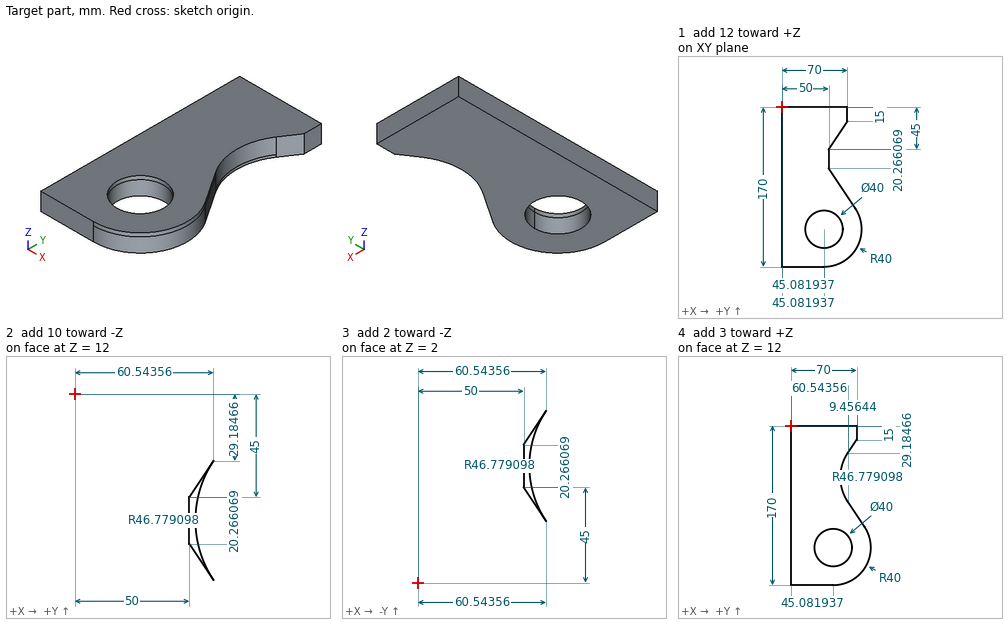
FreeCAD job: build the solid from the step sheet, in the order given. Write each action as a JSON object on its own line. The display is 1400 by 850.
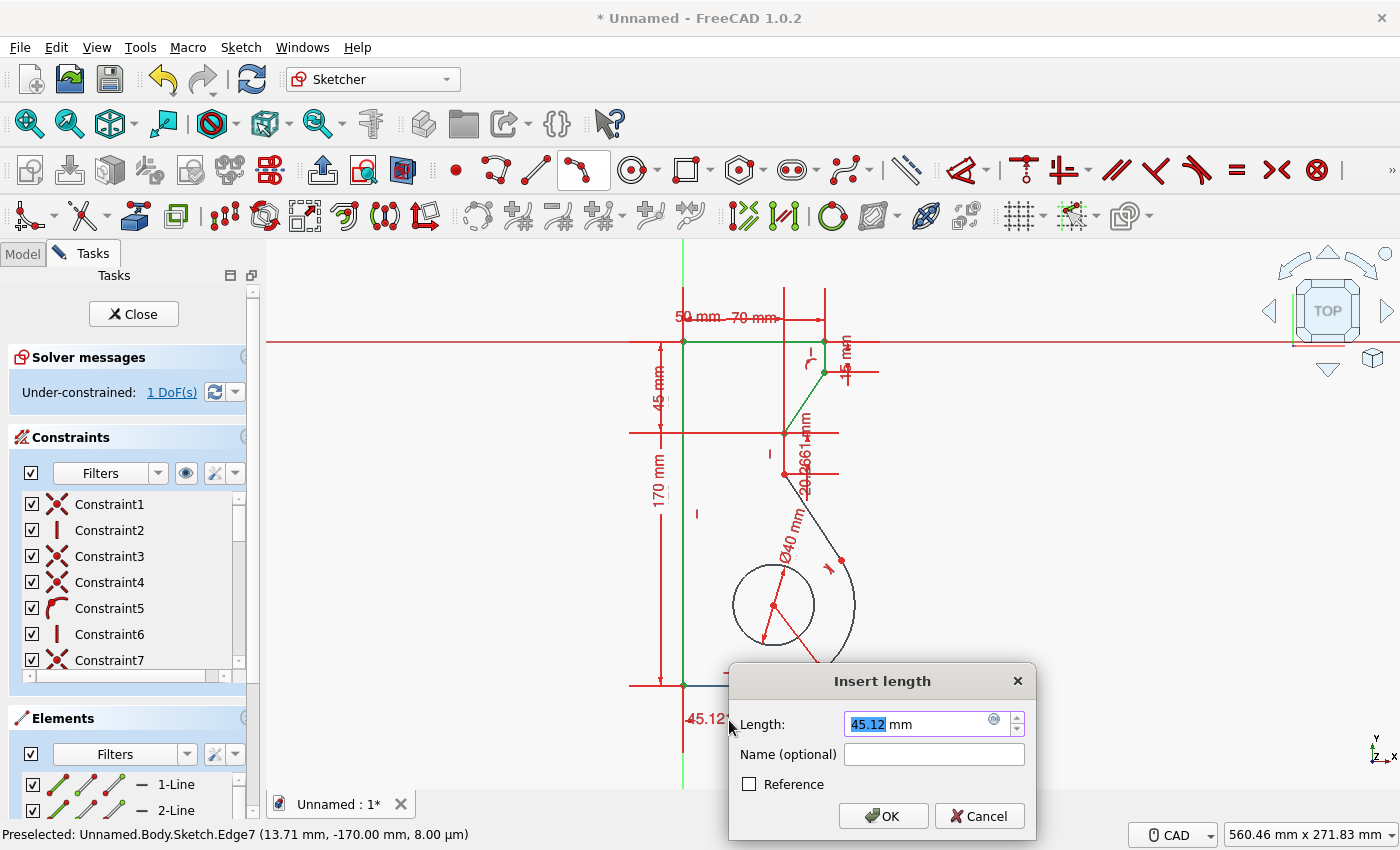
{"action": "type", "text": "45.081937"}
{"action": "key", "text": "Return"}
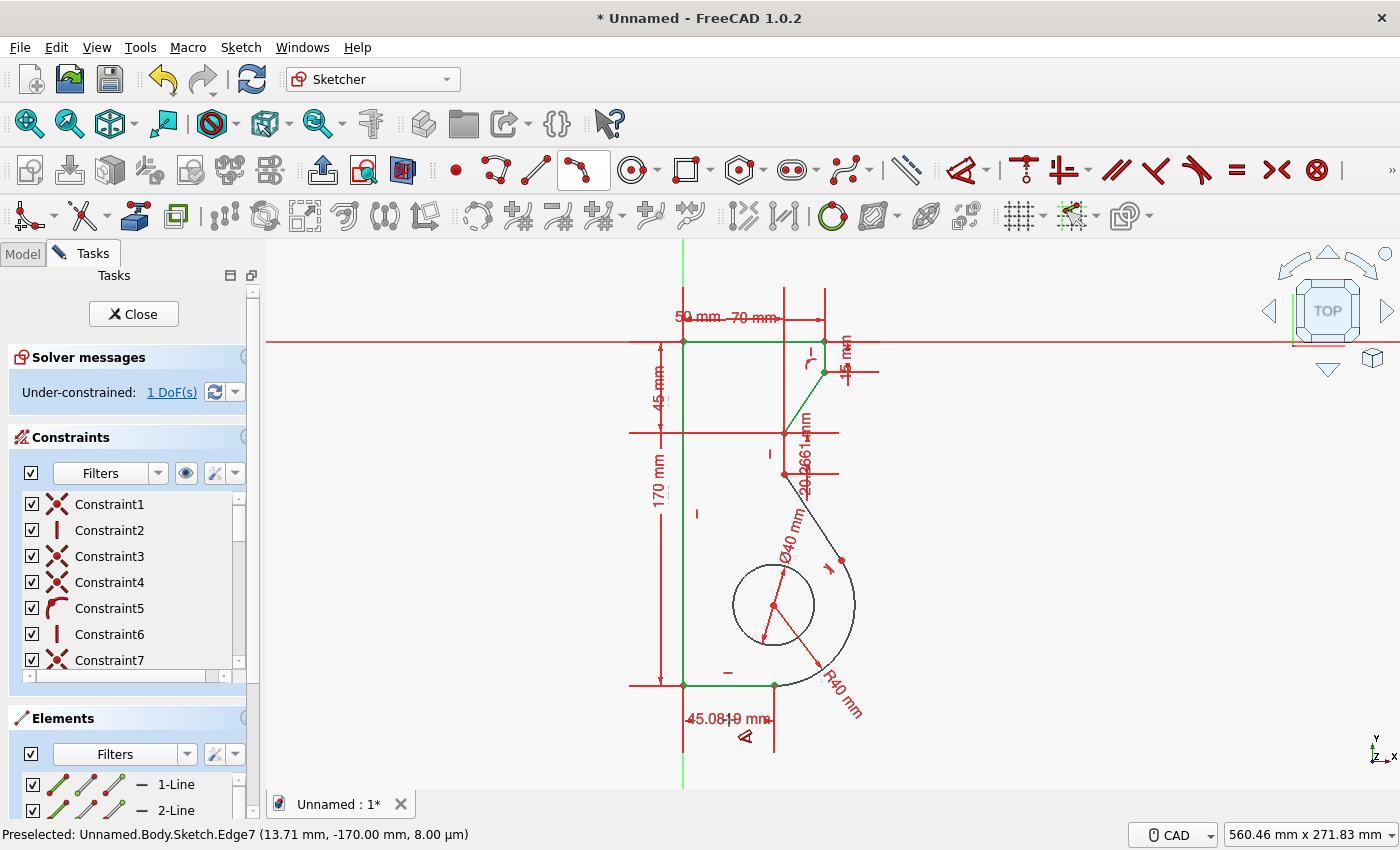
{"action": "left_click", "coordinate": [774, 605]}
{"action": "left_click", "coordinate": [728, 639]}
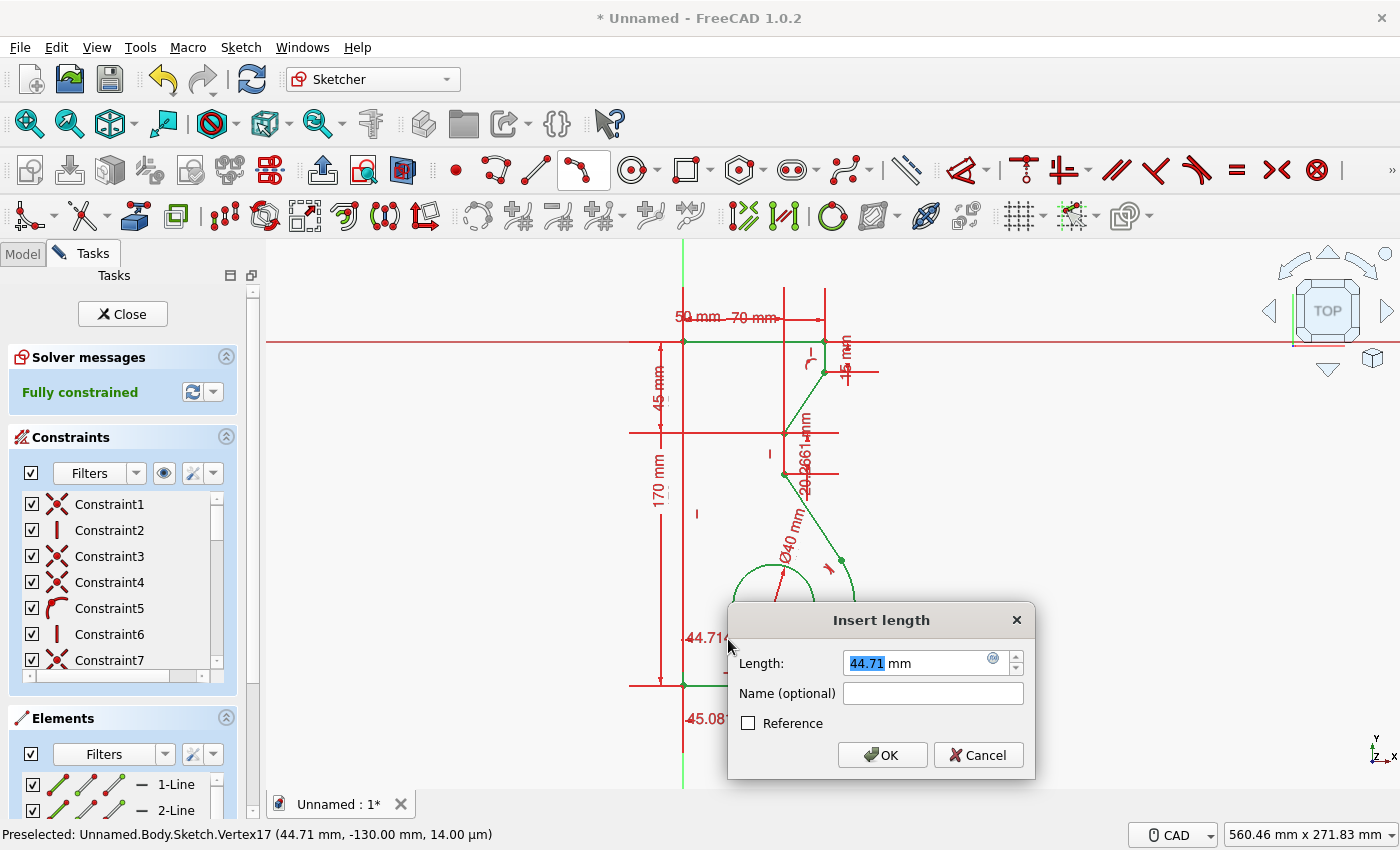
{"action": "type", "text": "45.081937"}
{"action": "key", "text": "Return"}
{"action": "key", "text": "Escape"}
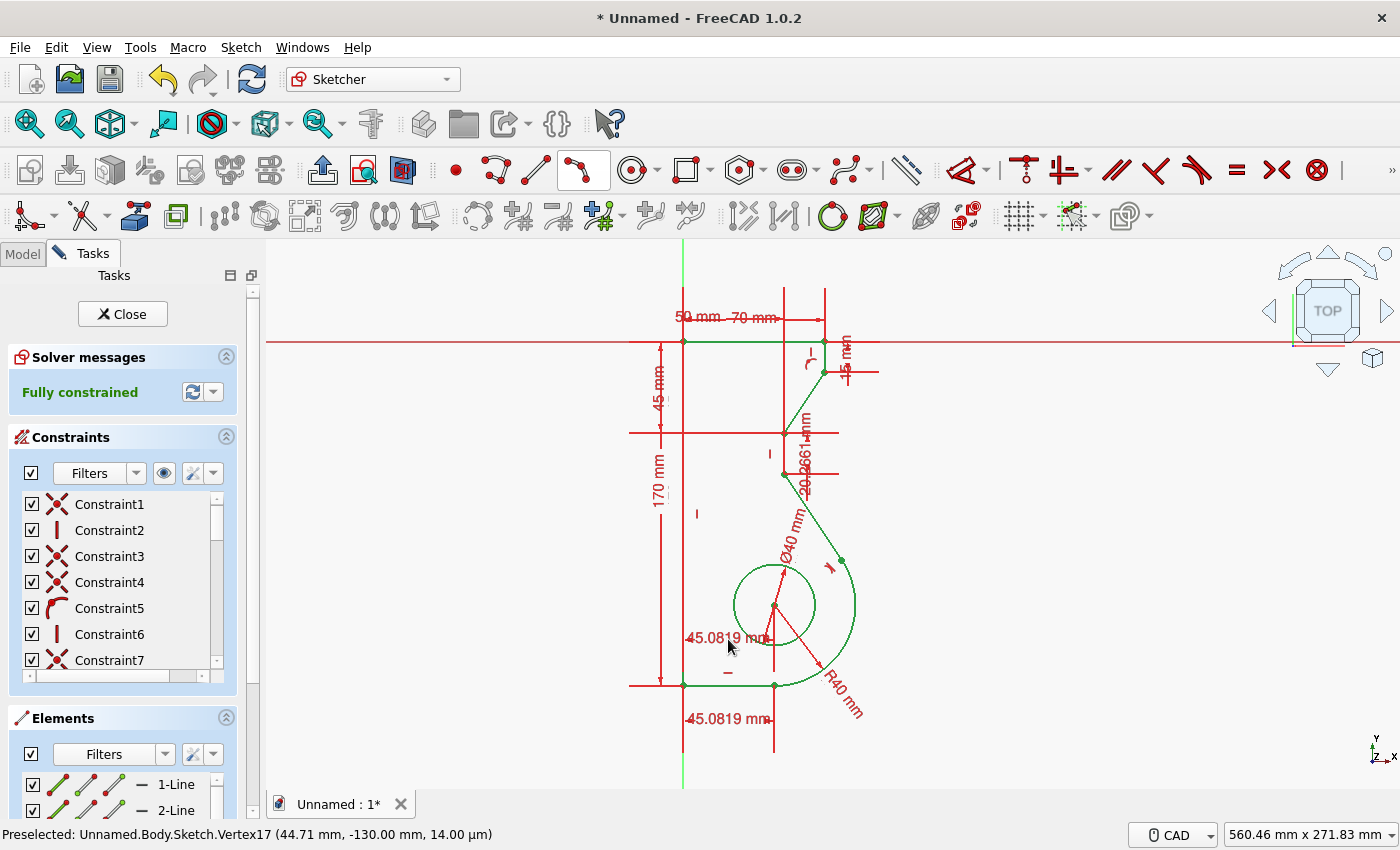
{"action": "left_click", "coordinate": [123, 314]}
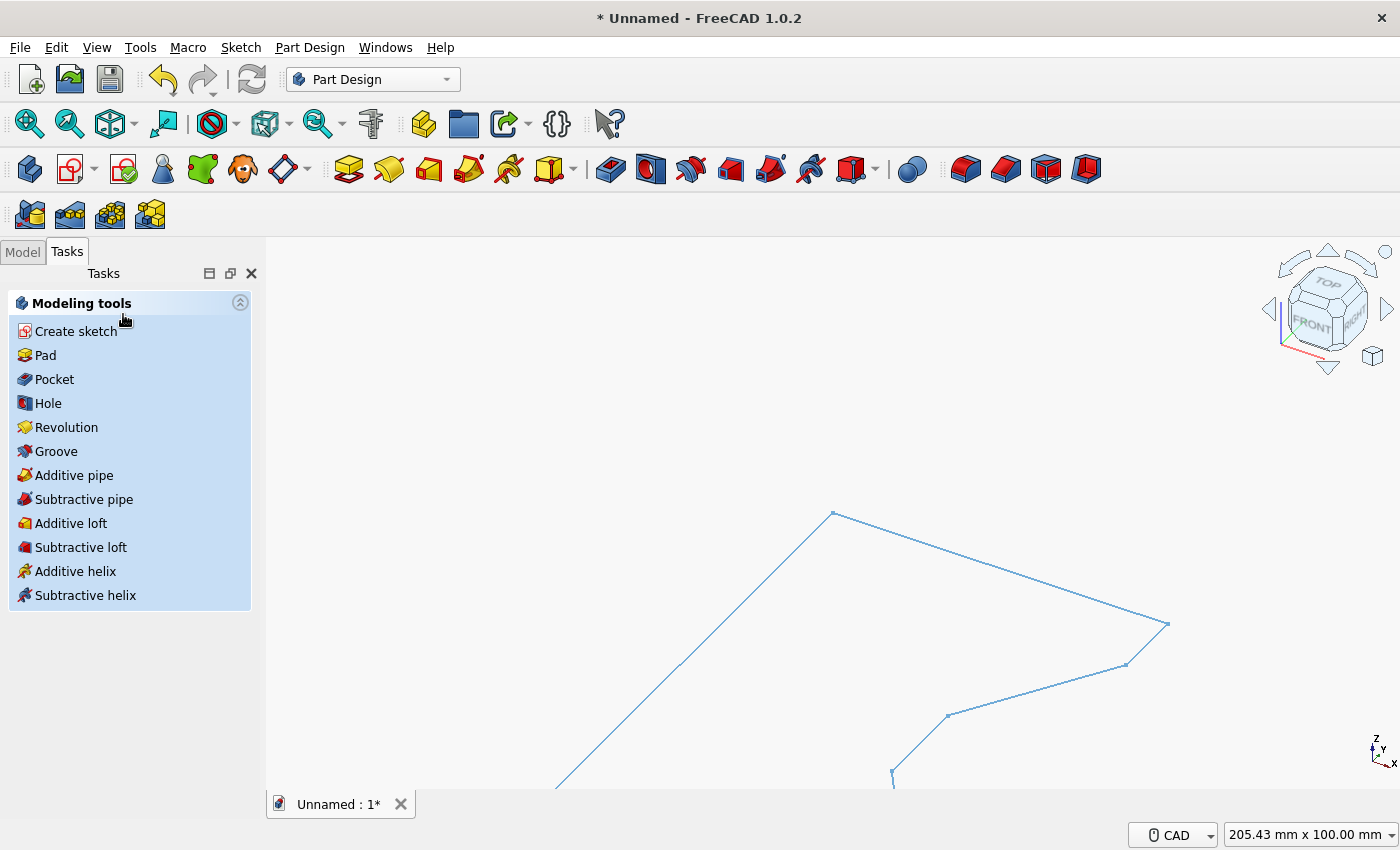
{"action": "left_click", "coordinate": [350, 170]}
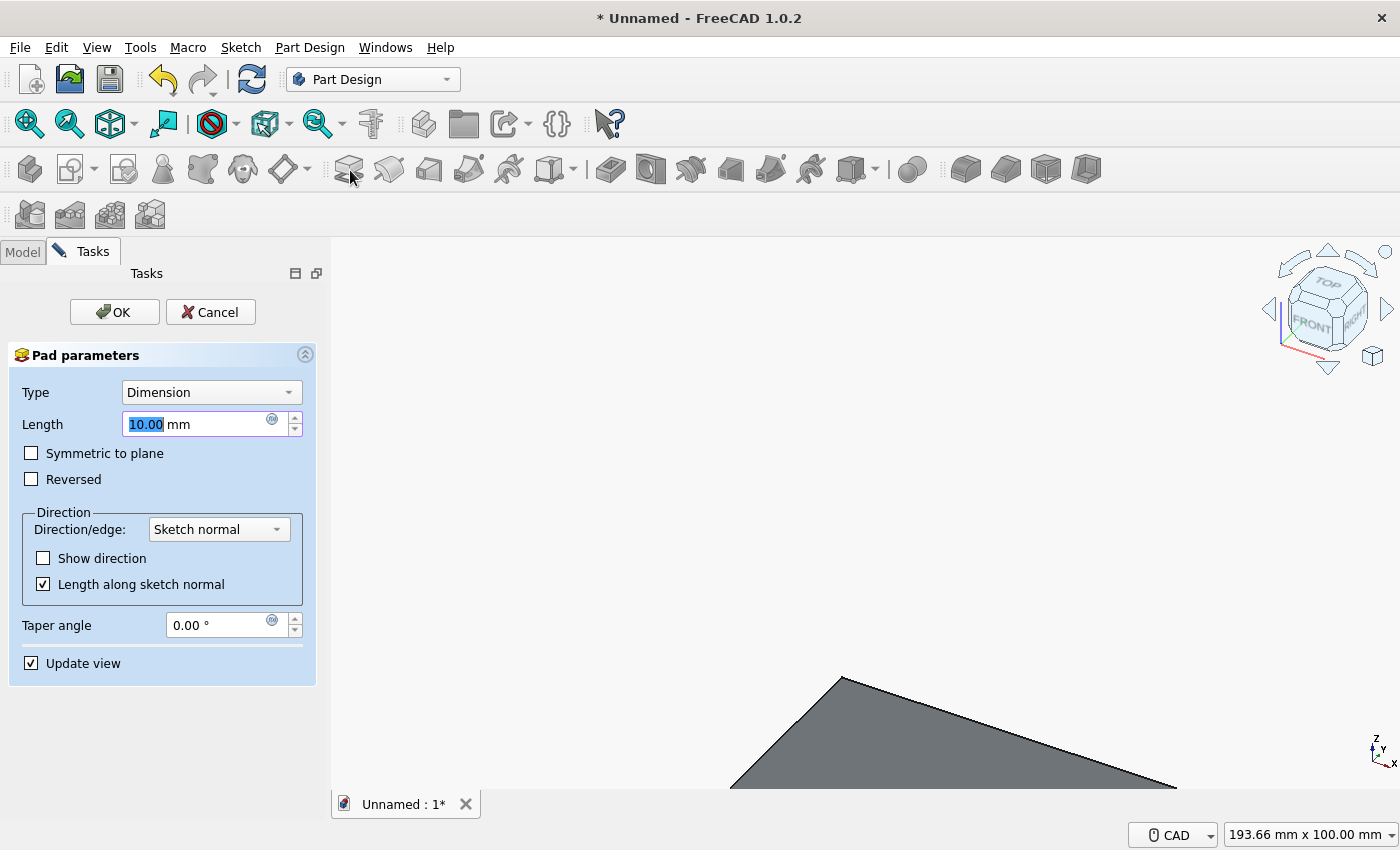
{"action": "type", "text": "12"}
{"action": "key", "text": "Tab"}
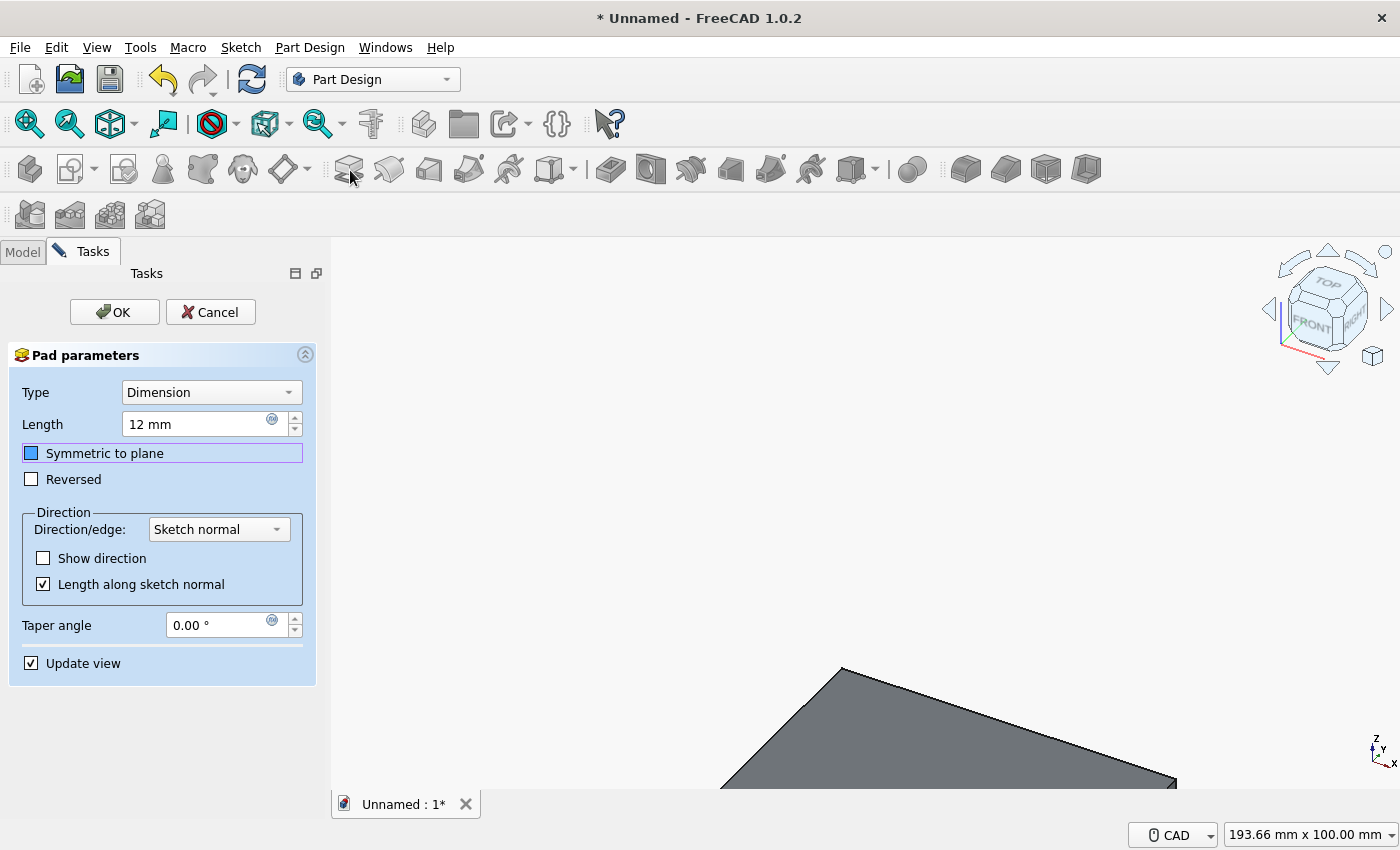
{"action": "left_click", "coordinate": [115, 312]}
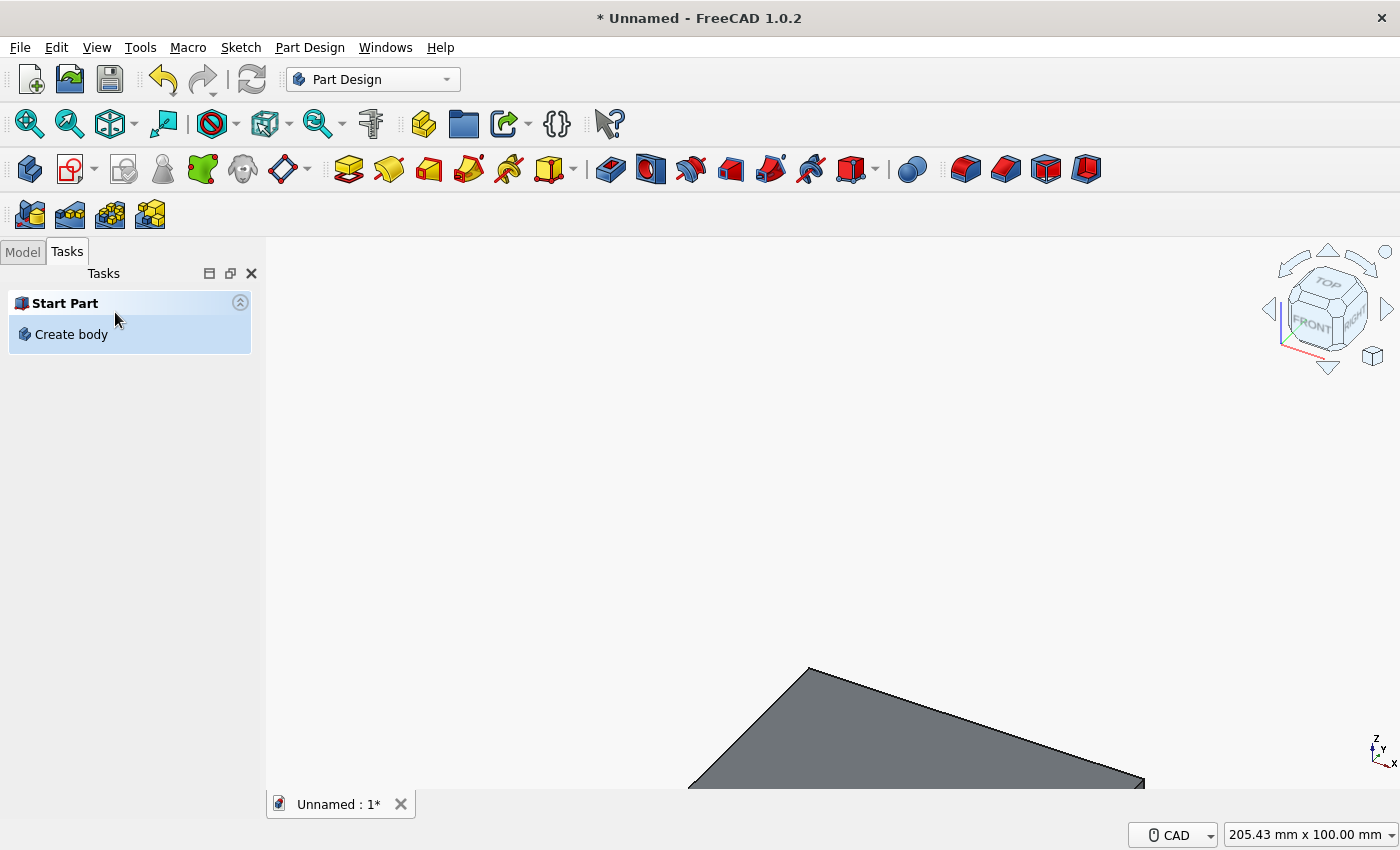
{"action": "left_click", "coordinate": [30, 124]}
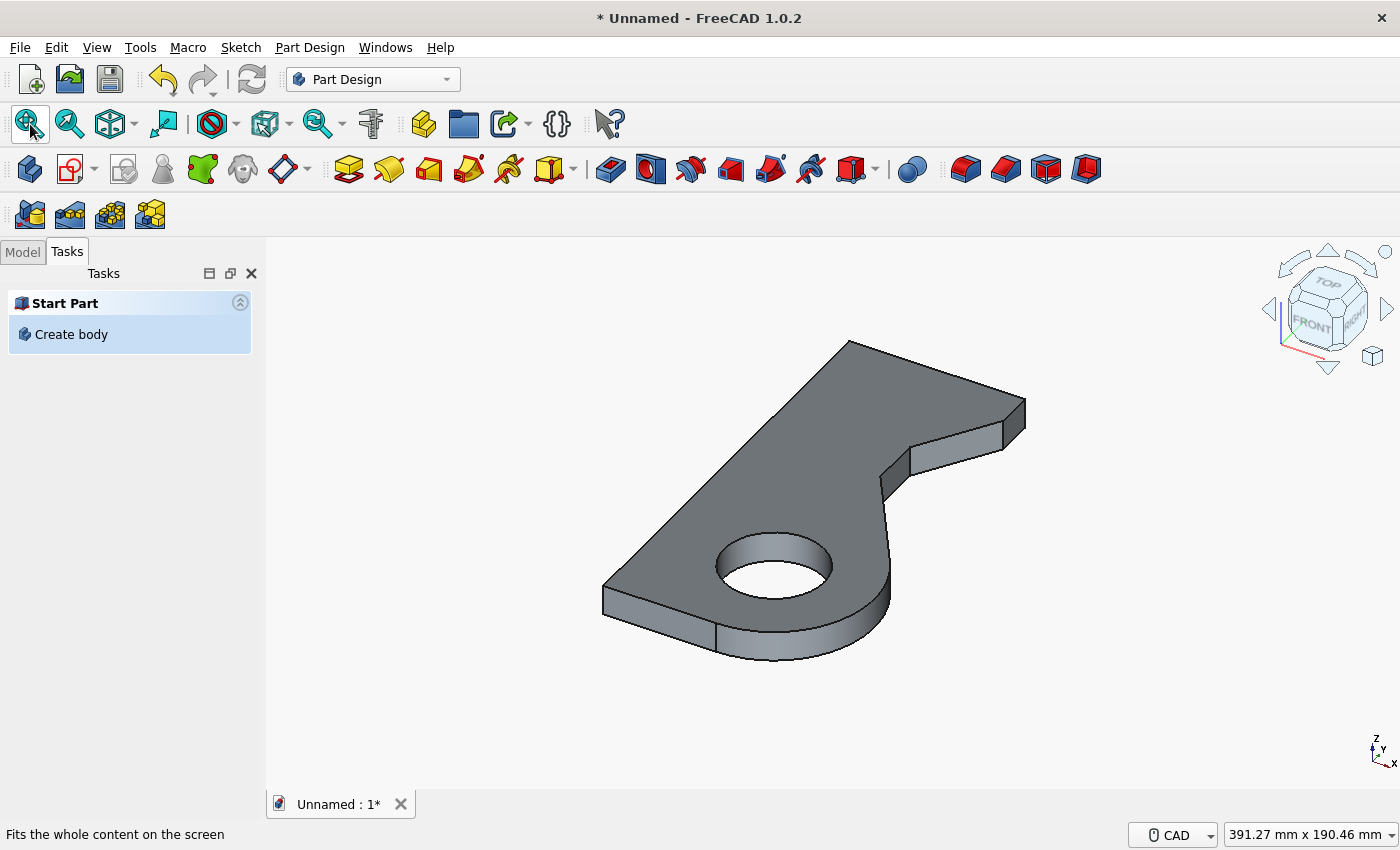
{"action": "left_click", "coordinate": [803, 488]}